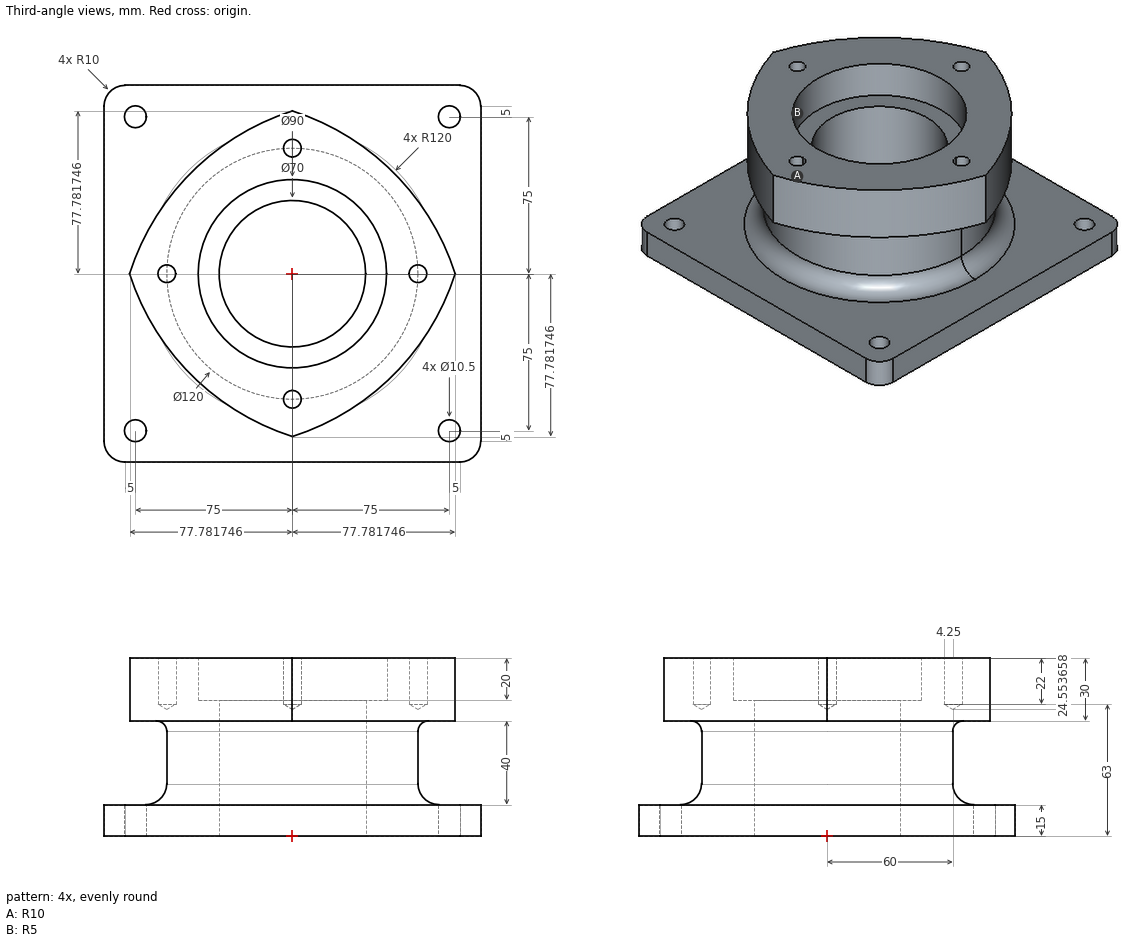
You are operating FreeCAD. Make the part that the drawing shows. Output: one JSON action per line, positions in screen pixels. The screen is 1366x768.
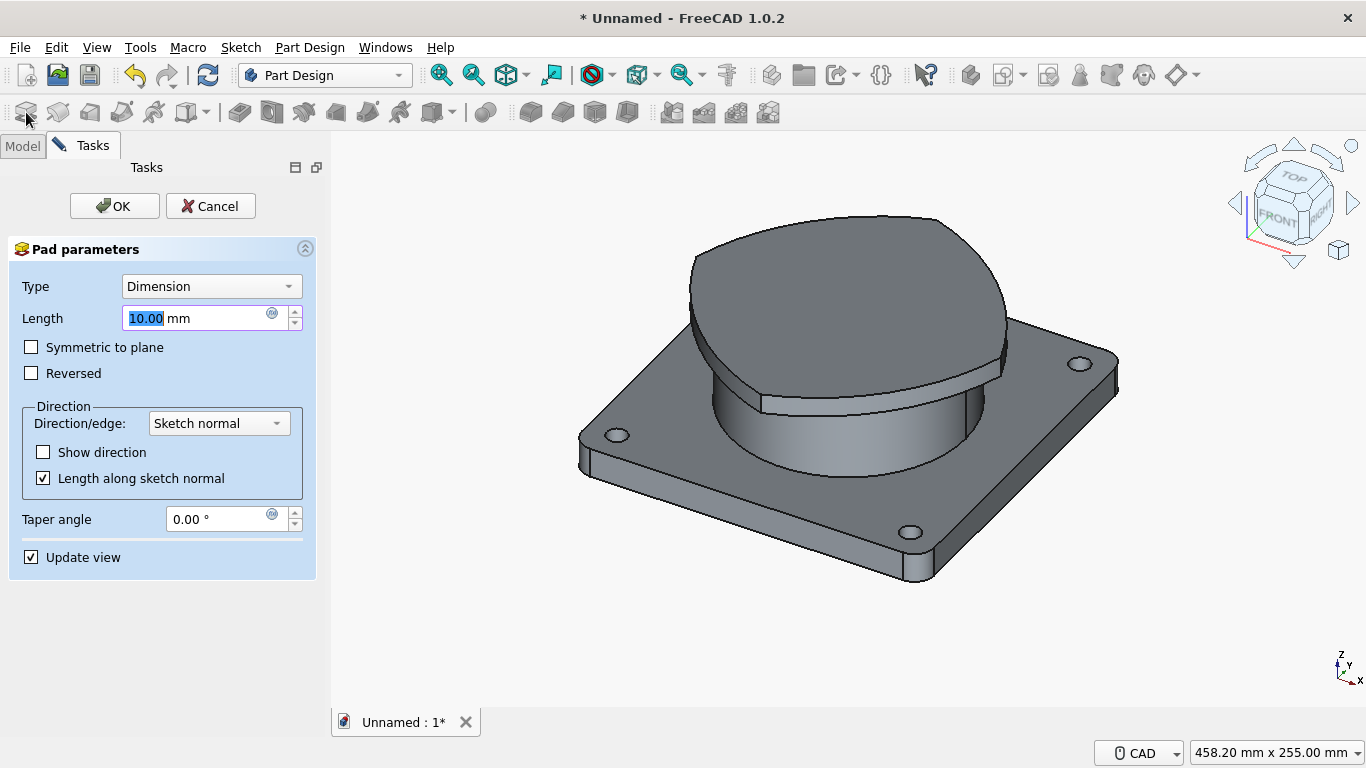
{"action": "type", "text": "30"}
{"action": "key", "text": "Tab"}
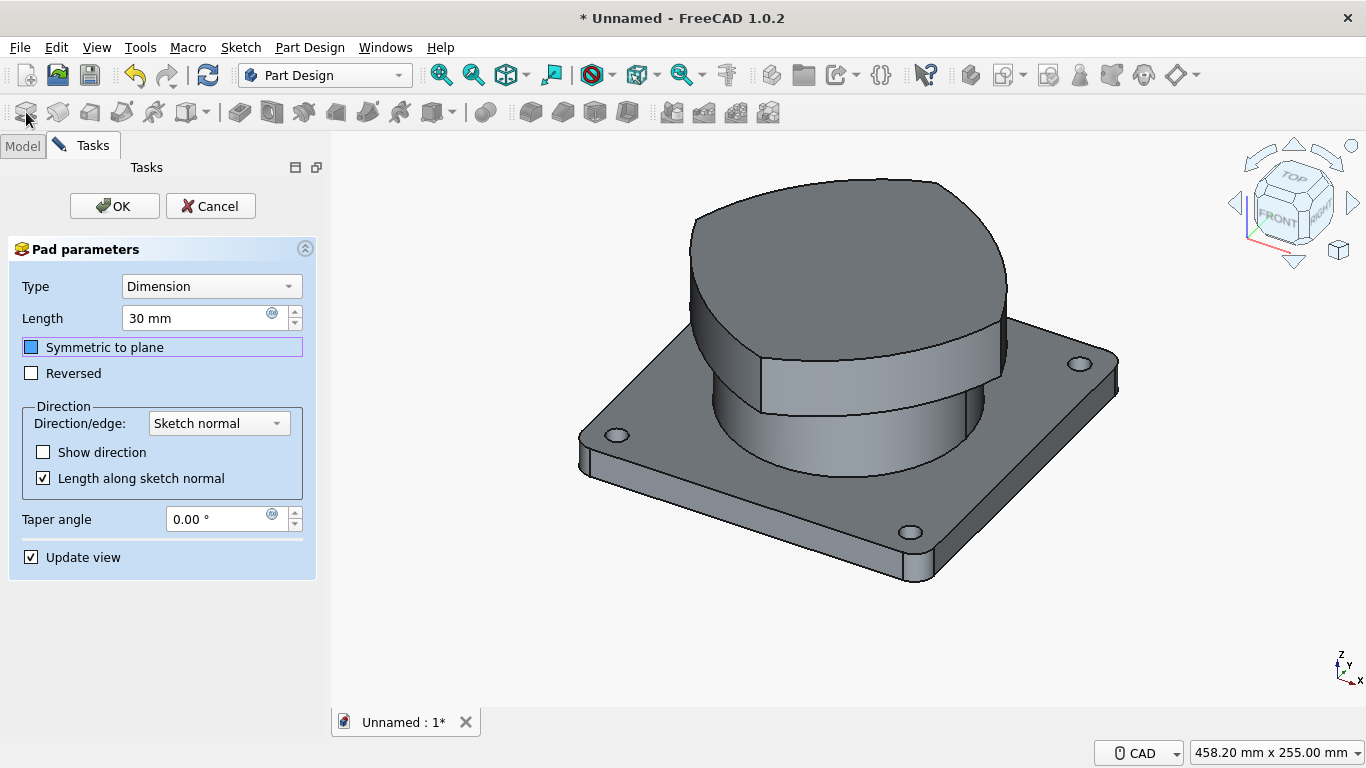
{"action": "left_click", "coordinate": [115, 206]}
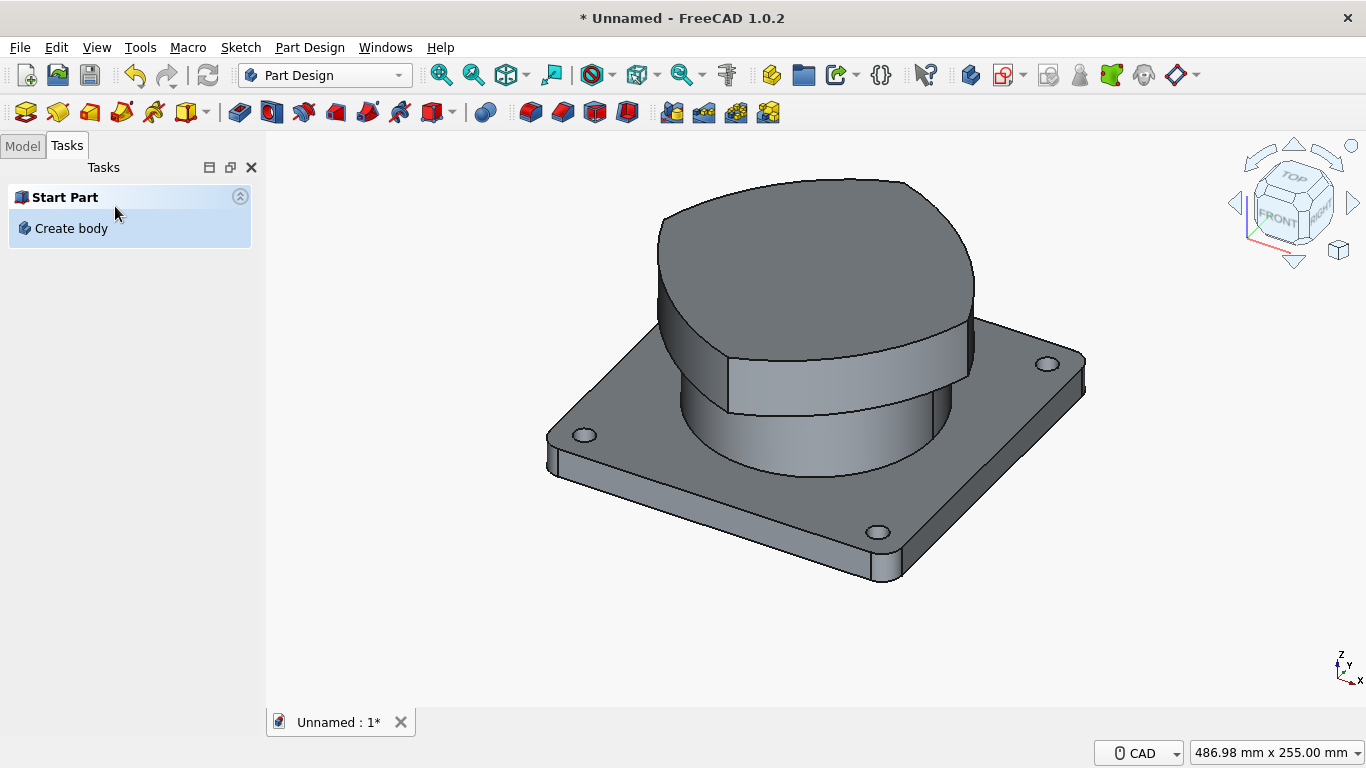
{"action": "left_click", "coordinate": [442, 76]}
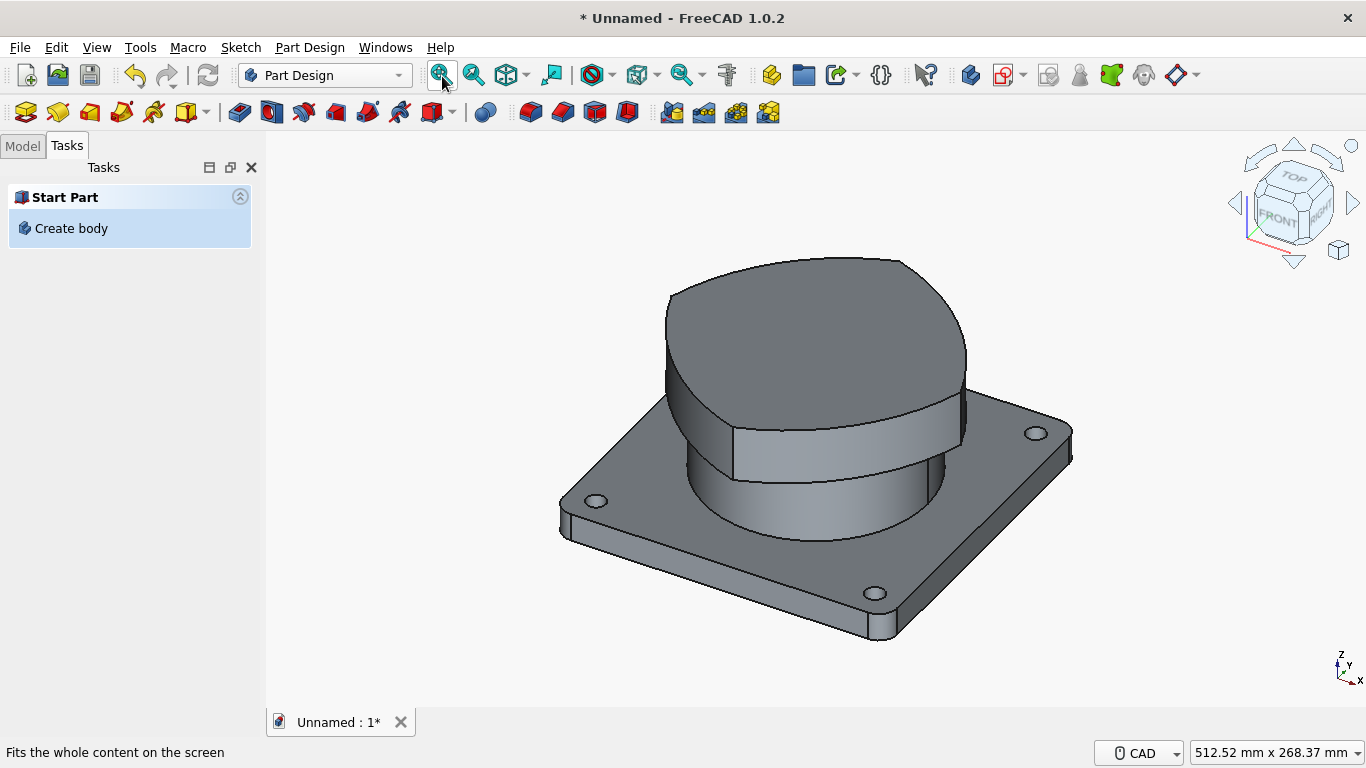
{"action": "left_click", "coordinate": [1004, 76]}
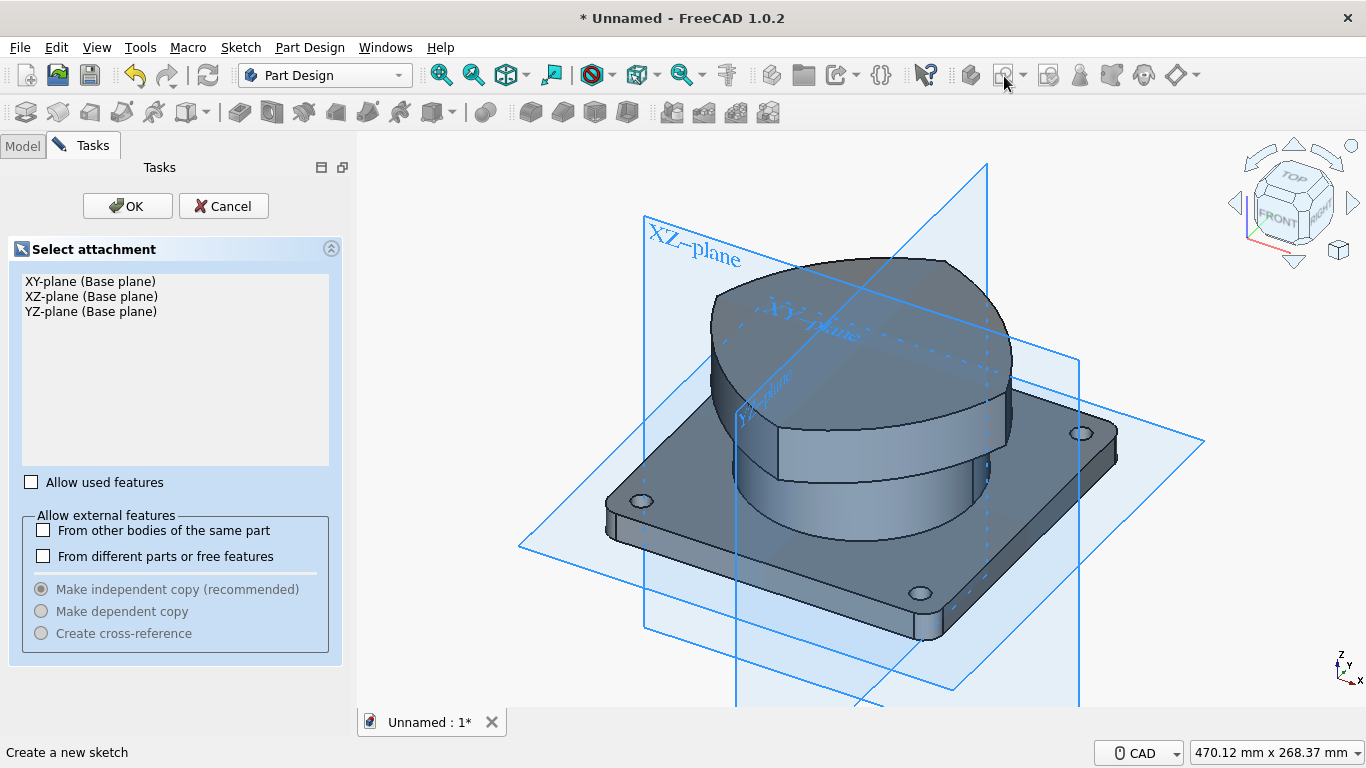
{"action": "left_click", "coordinate": [82, 312]}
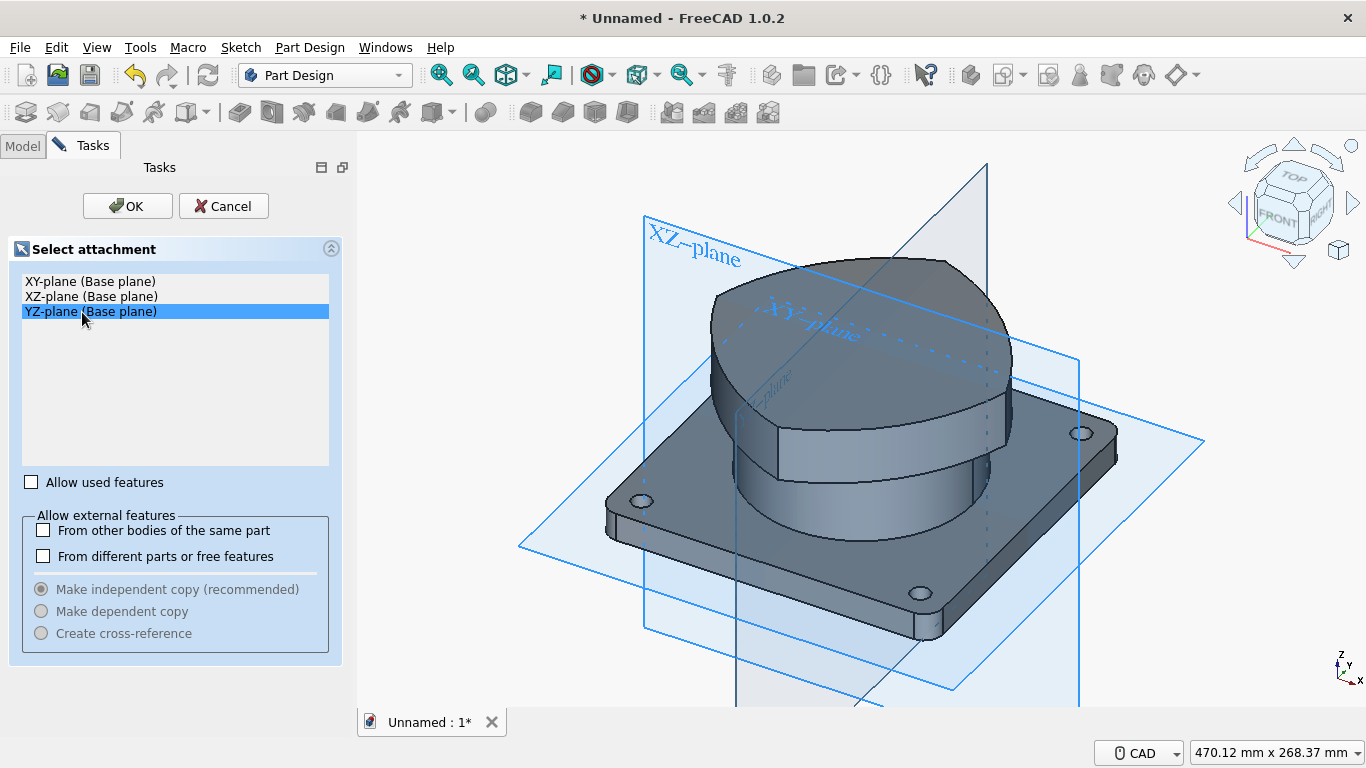
{"action": "left_click", "coordinate": [128, 206]}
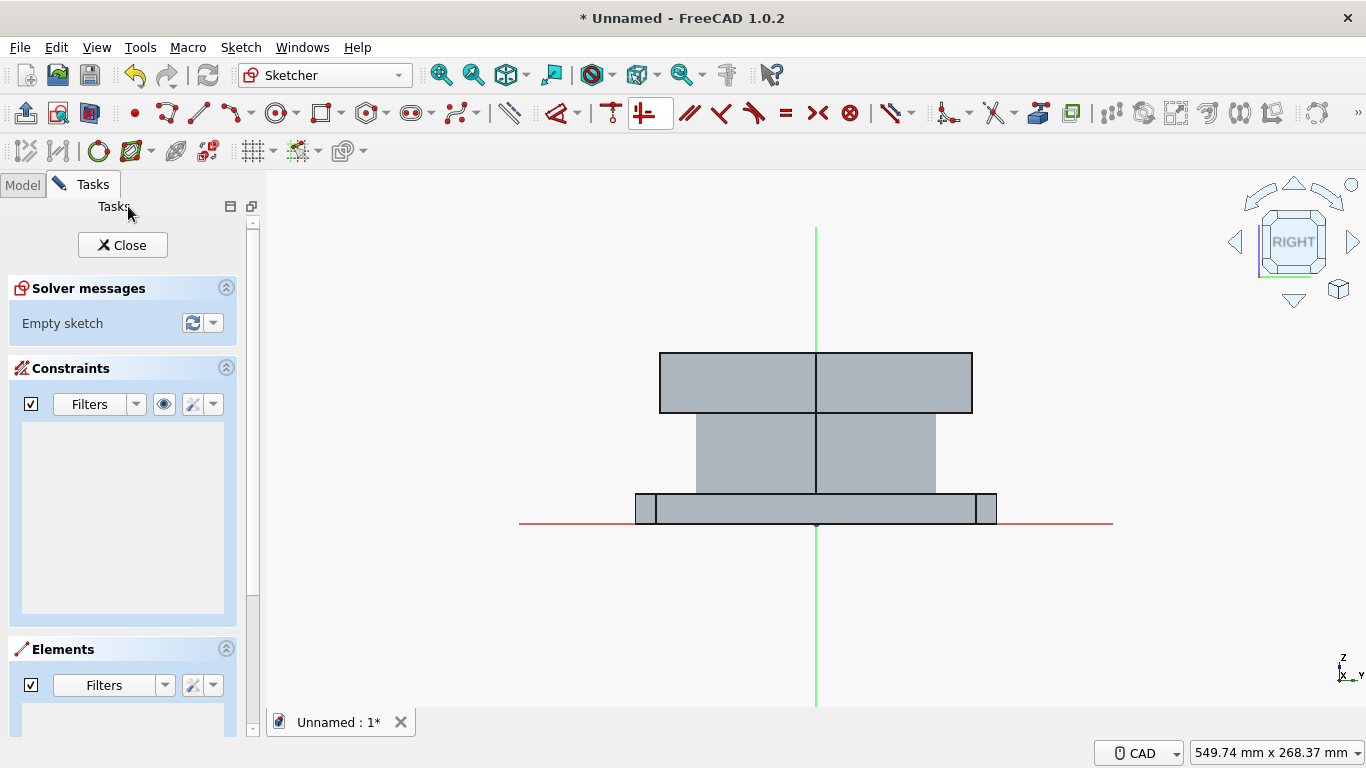
{"action": "left_click", "coordinate": [90, 114]}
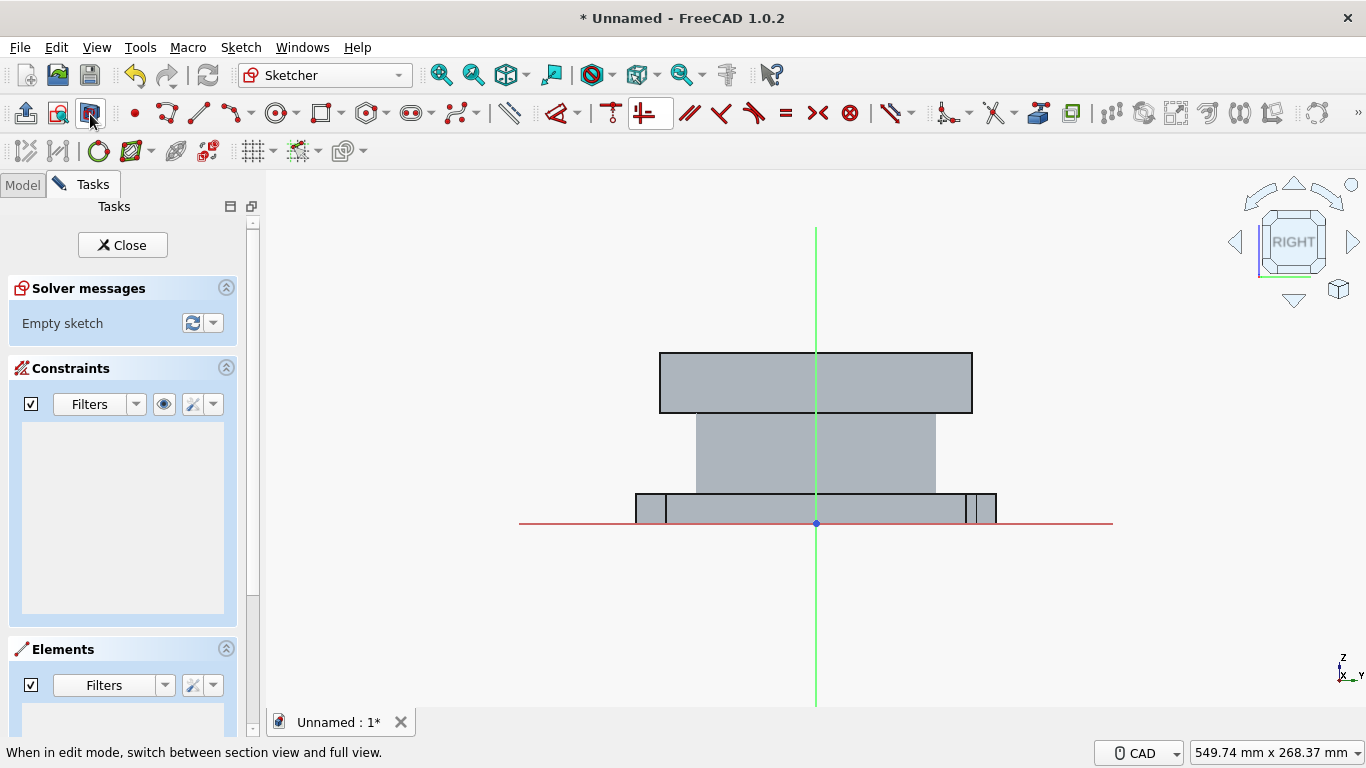
{"action": "scroll", "coordinate": [1032, 438], "scroll_direction": "up", "scroll_amount": 3}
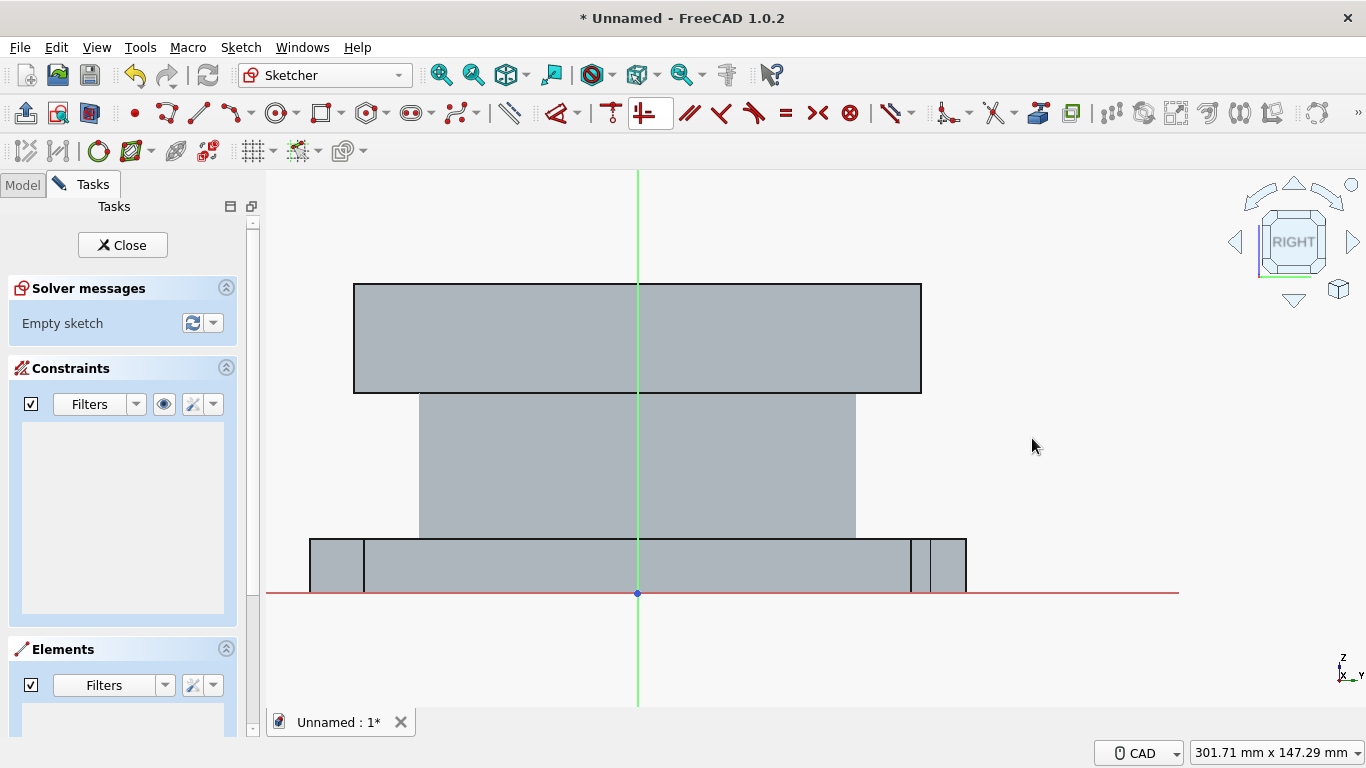
{"action": "left_click", "coordinate": [168, 114]}